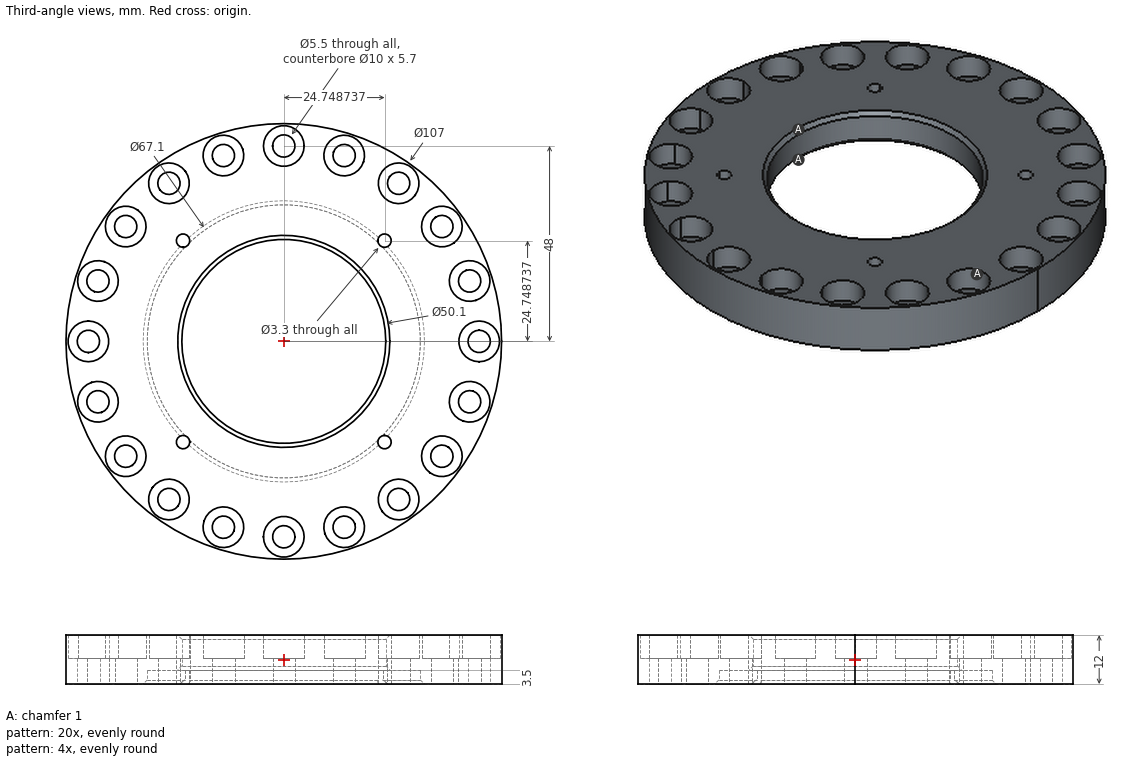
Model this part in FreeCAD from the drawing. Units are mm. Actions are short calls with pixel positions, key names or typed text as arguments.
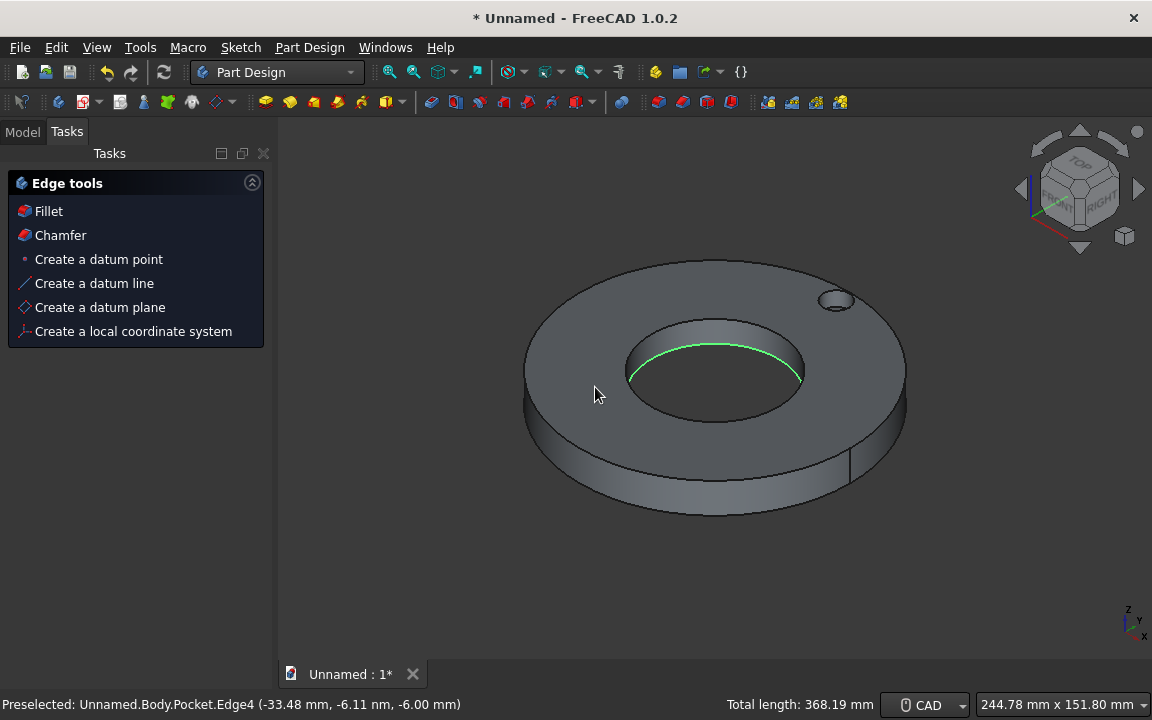
click(652, 333, ctrl)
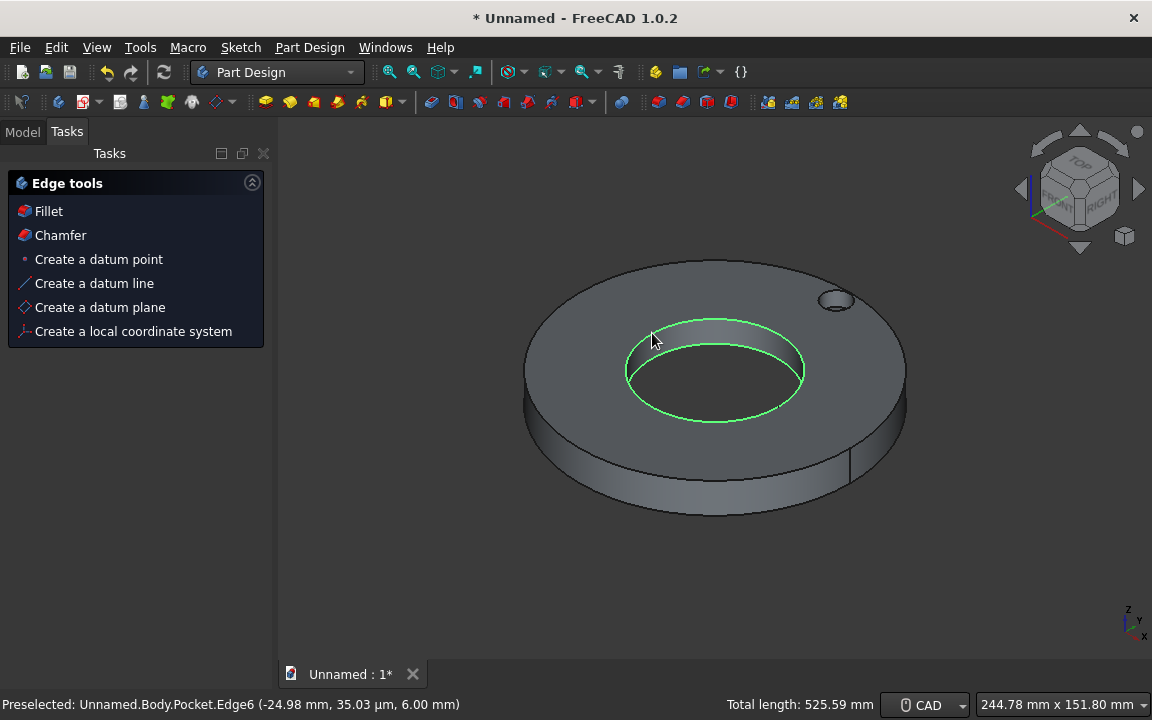
click(684, 102)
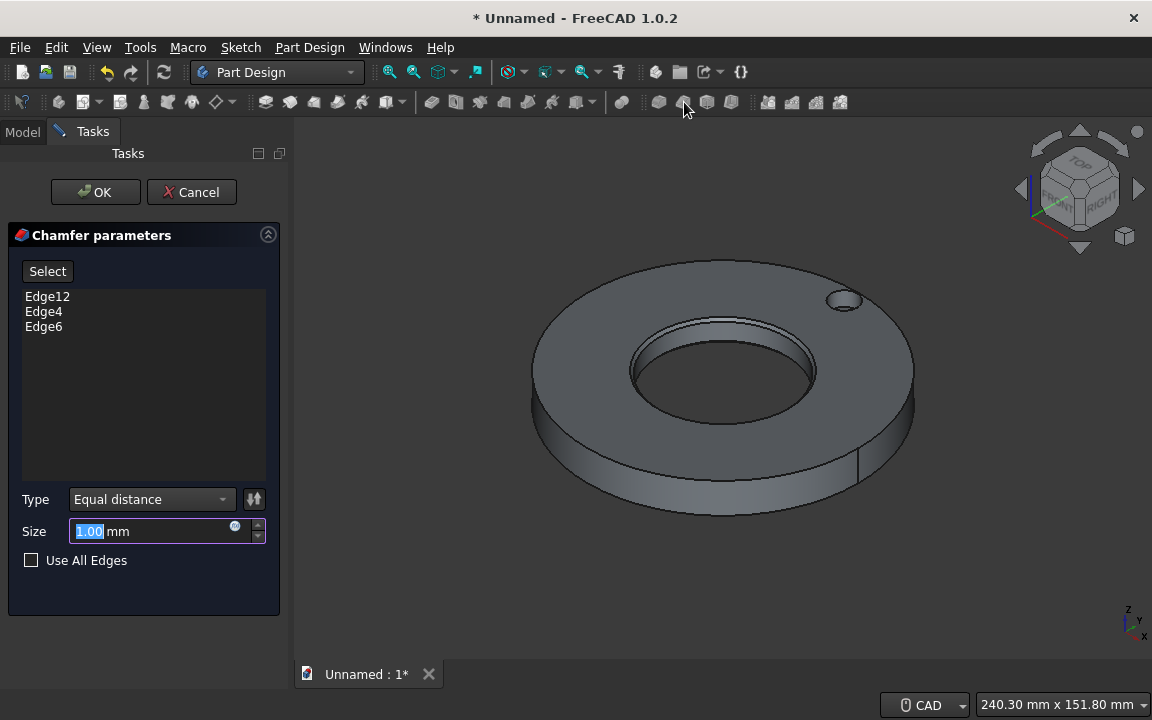
text(1)
key(Tab)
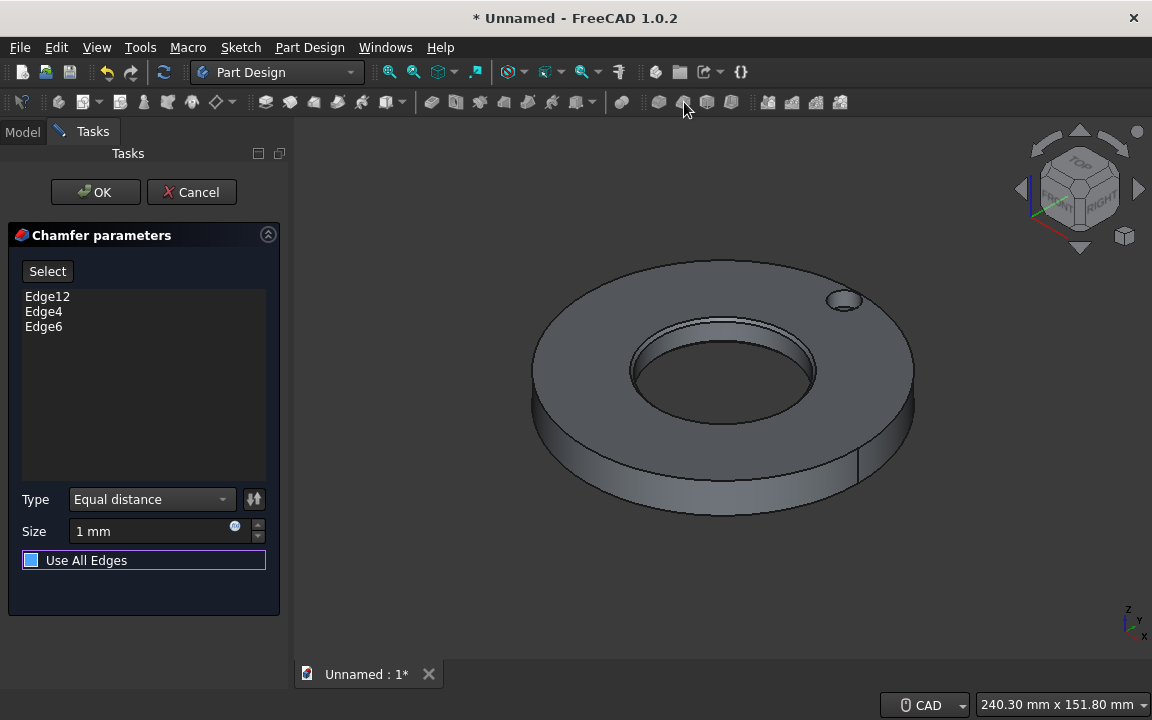
click(96, 192)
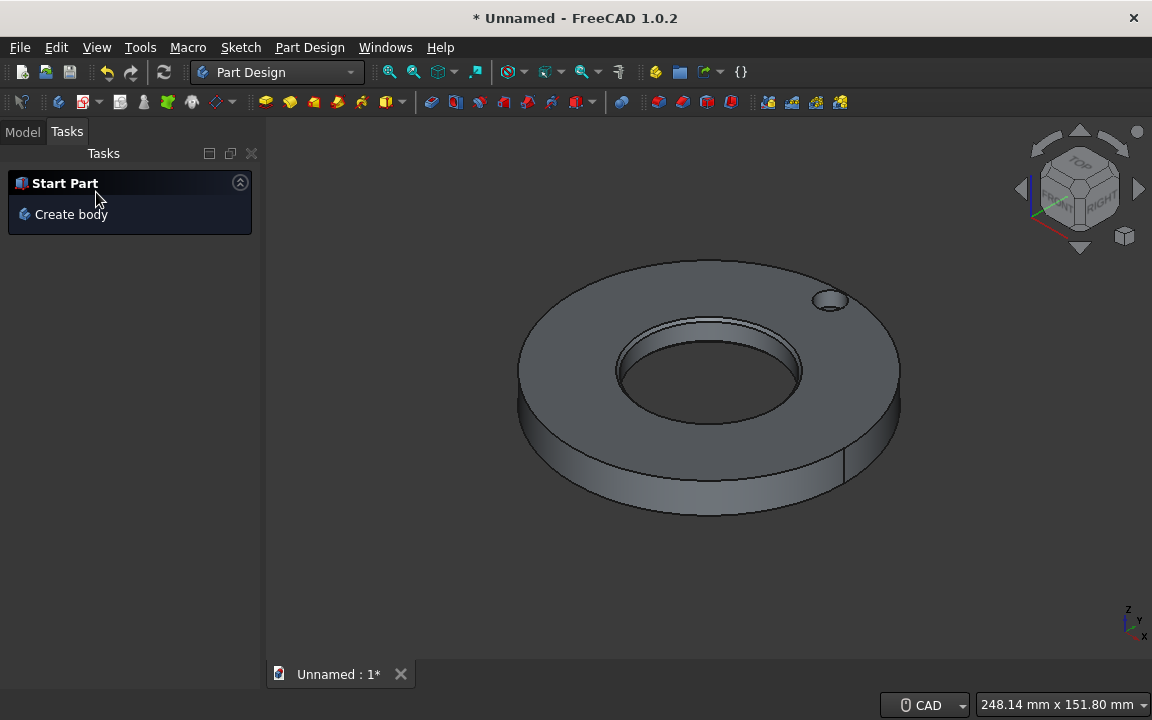
click(863, 370)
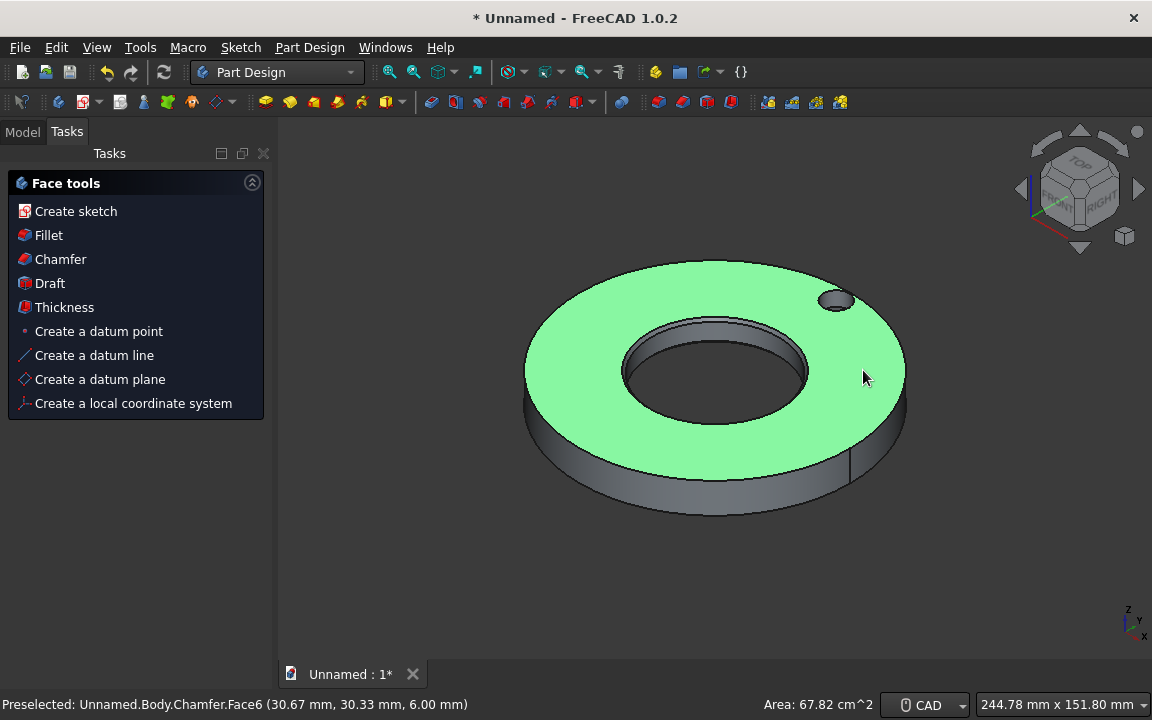
click(84, 102)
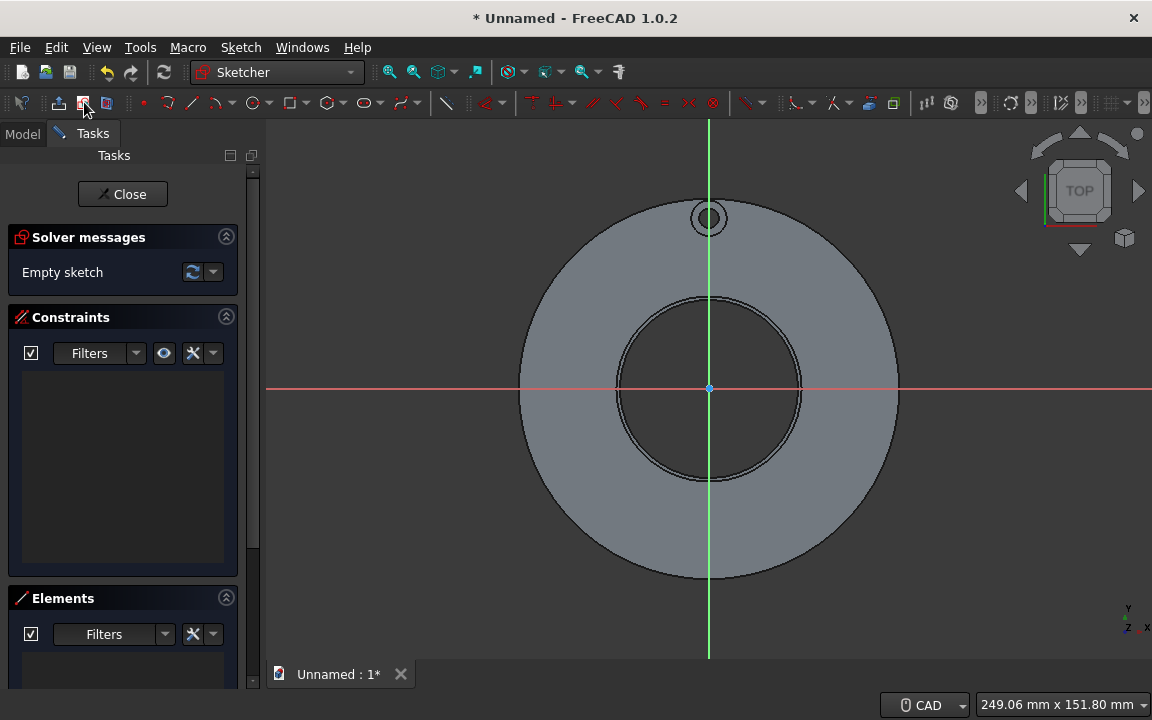
scroll(805, 296, up, 15)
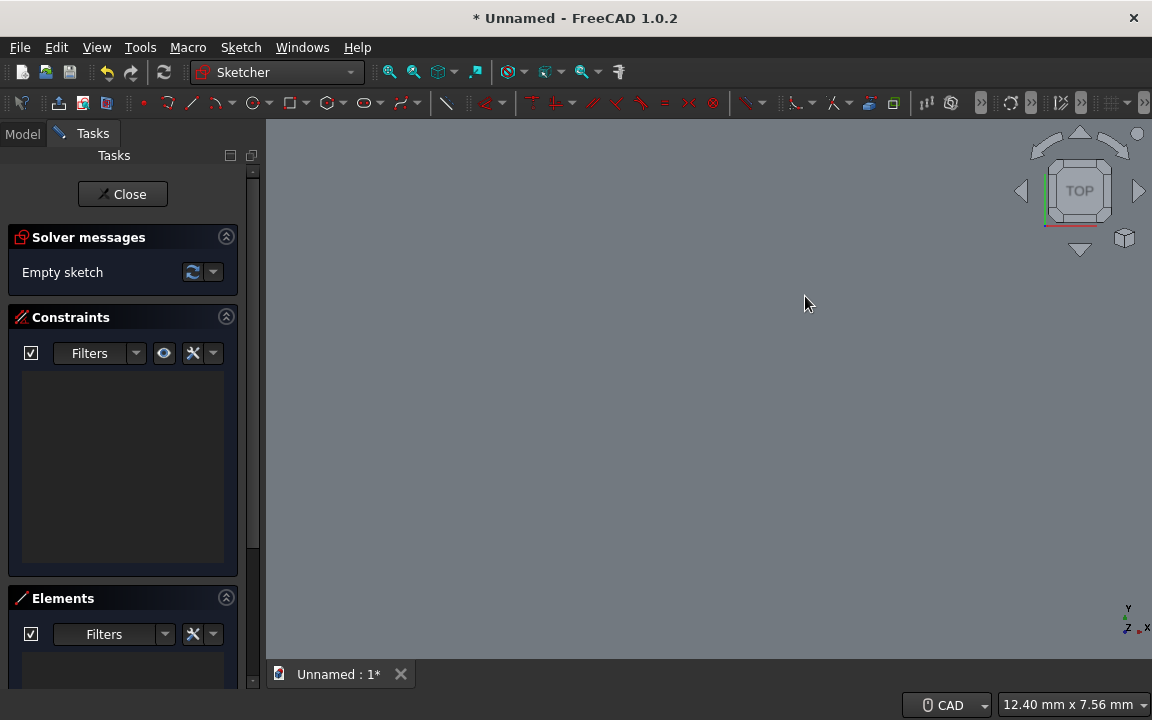
scroll(619, 390, up, 2)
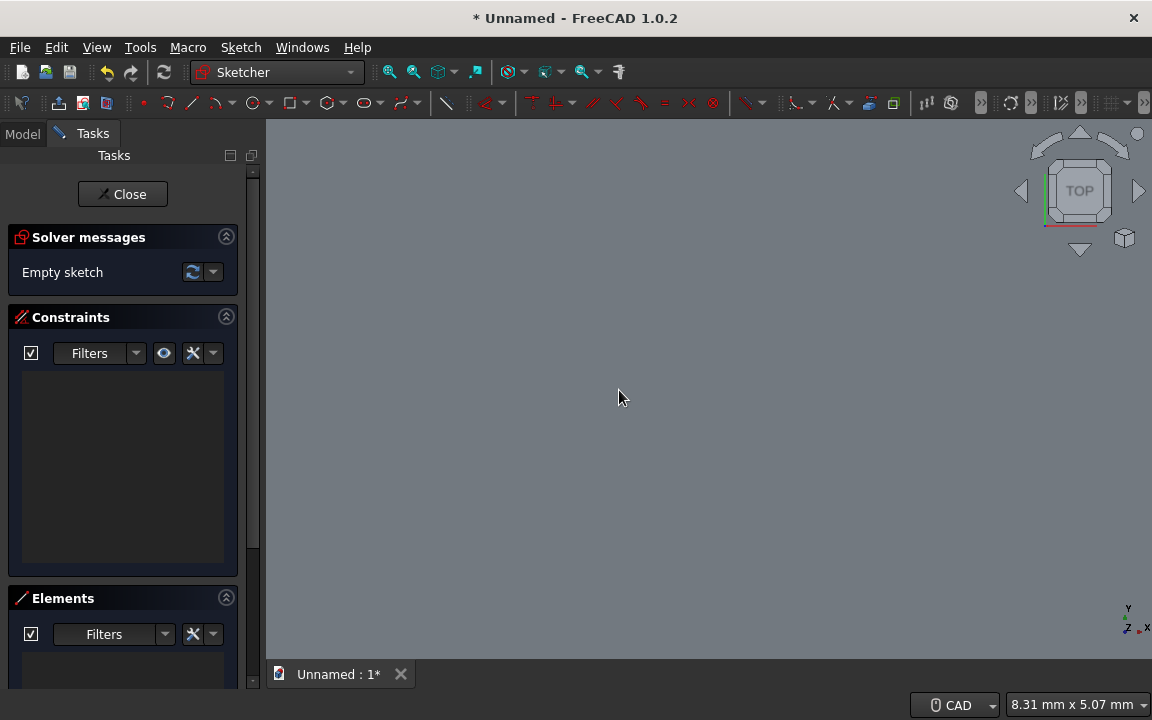
click(254, 104)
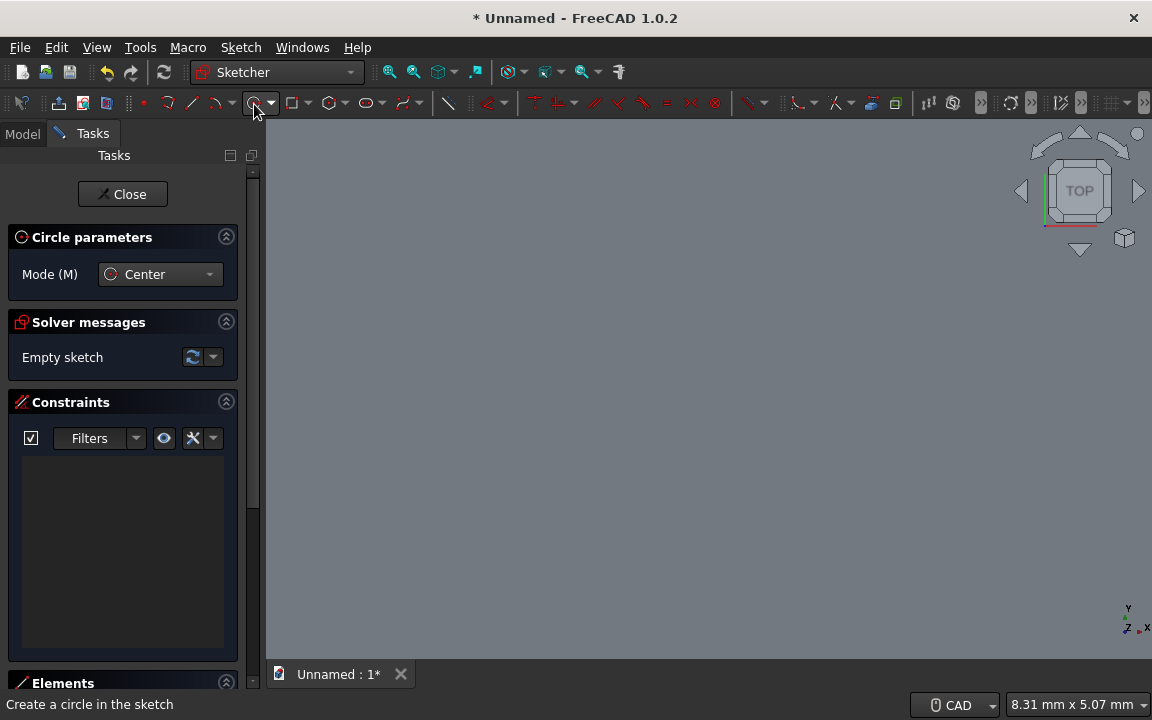
click(640, 389)
click(765, 264)
key(Escape)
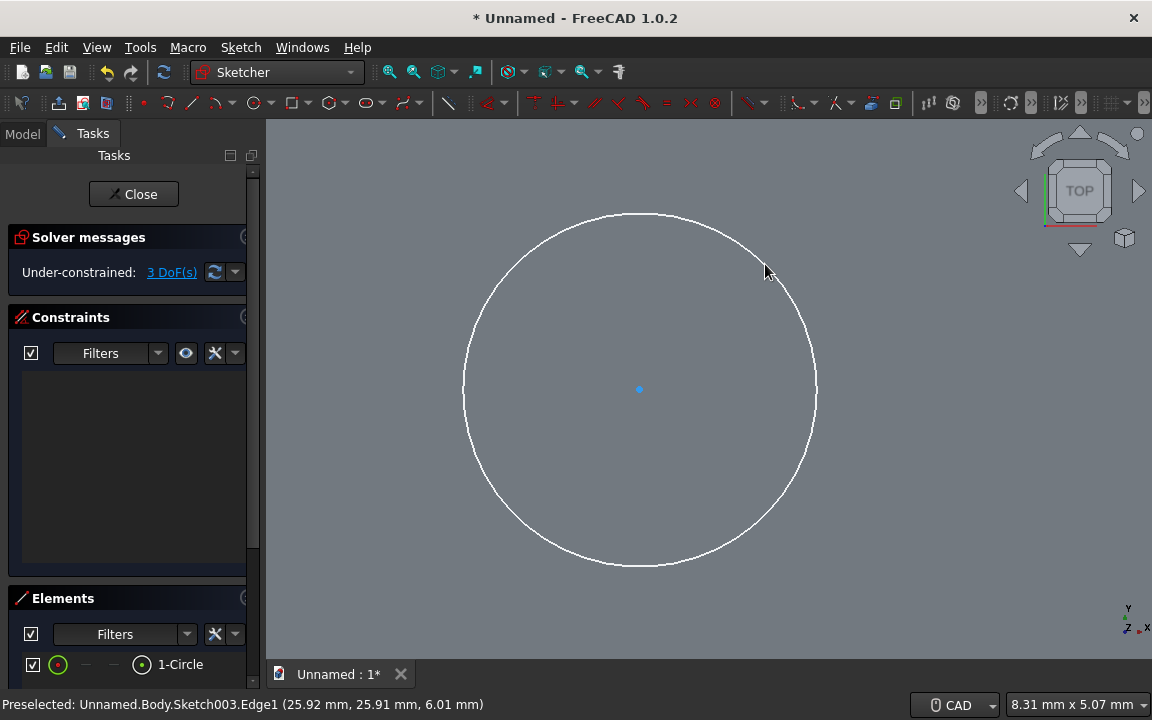
click(488, 104)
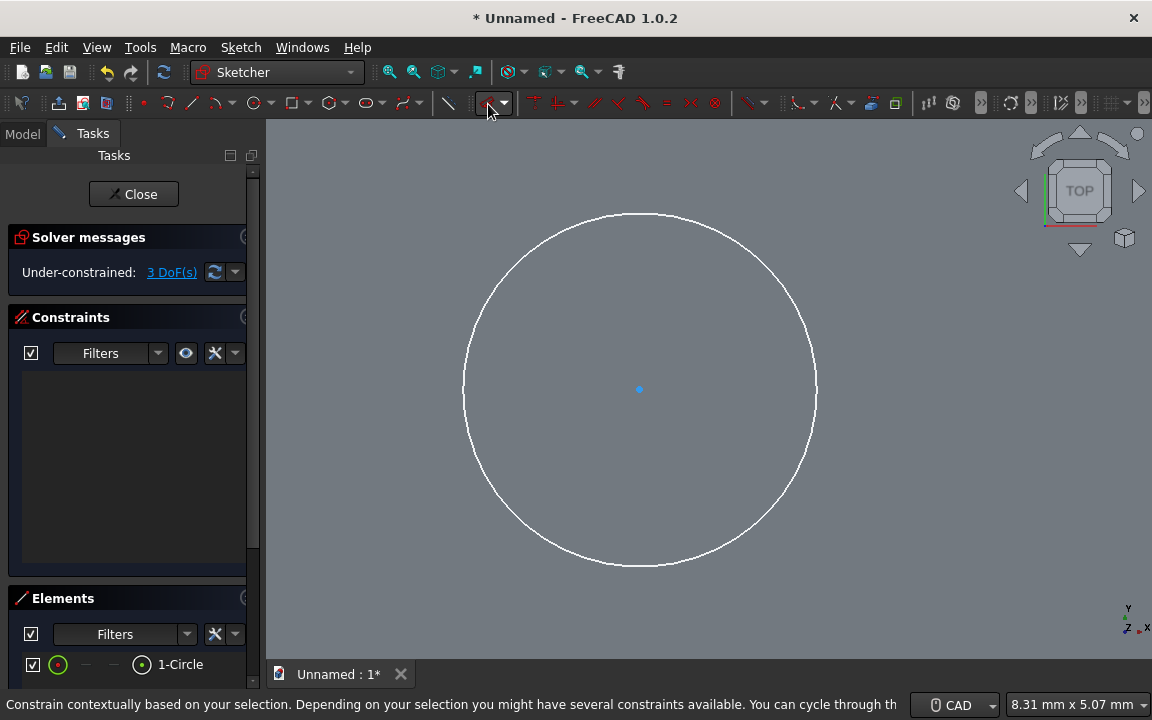
click(765, 265)
click(788, 242)